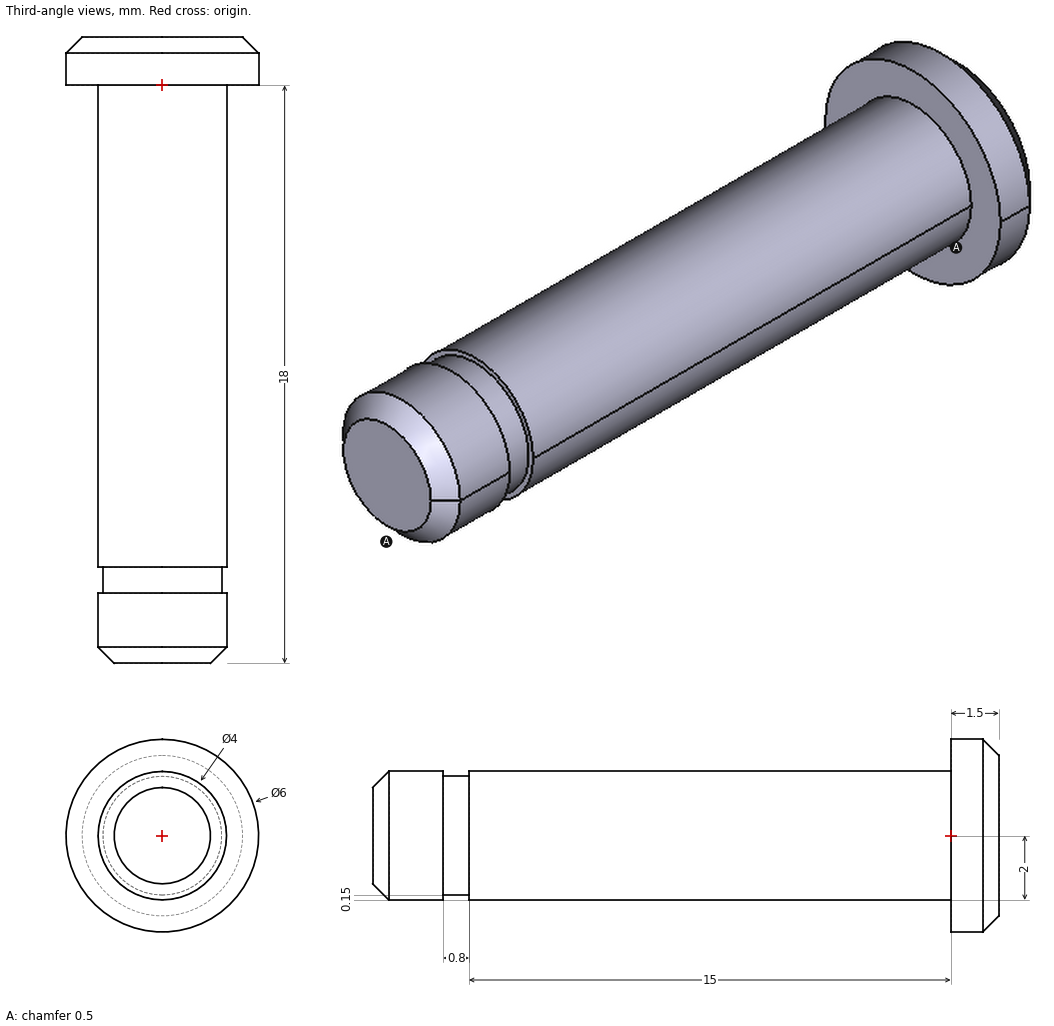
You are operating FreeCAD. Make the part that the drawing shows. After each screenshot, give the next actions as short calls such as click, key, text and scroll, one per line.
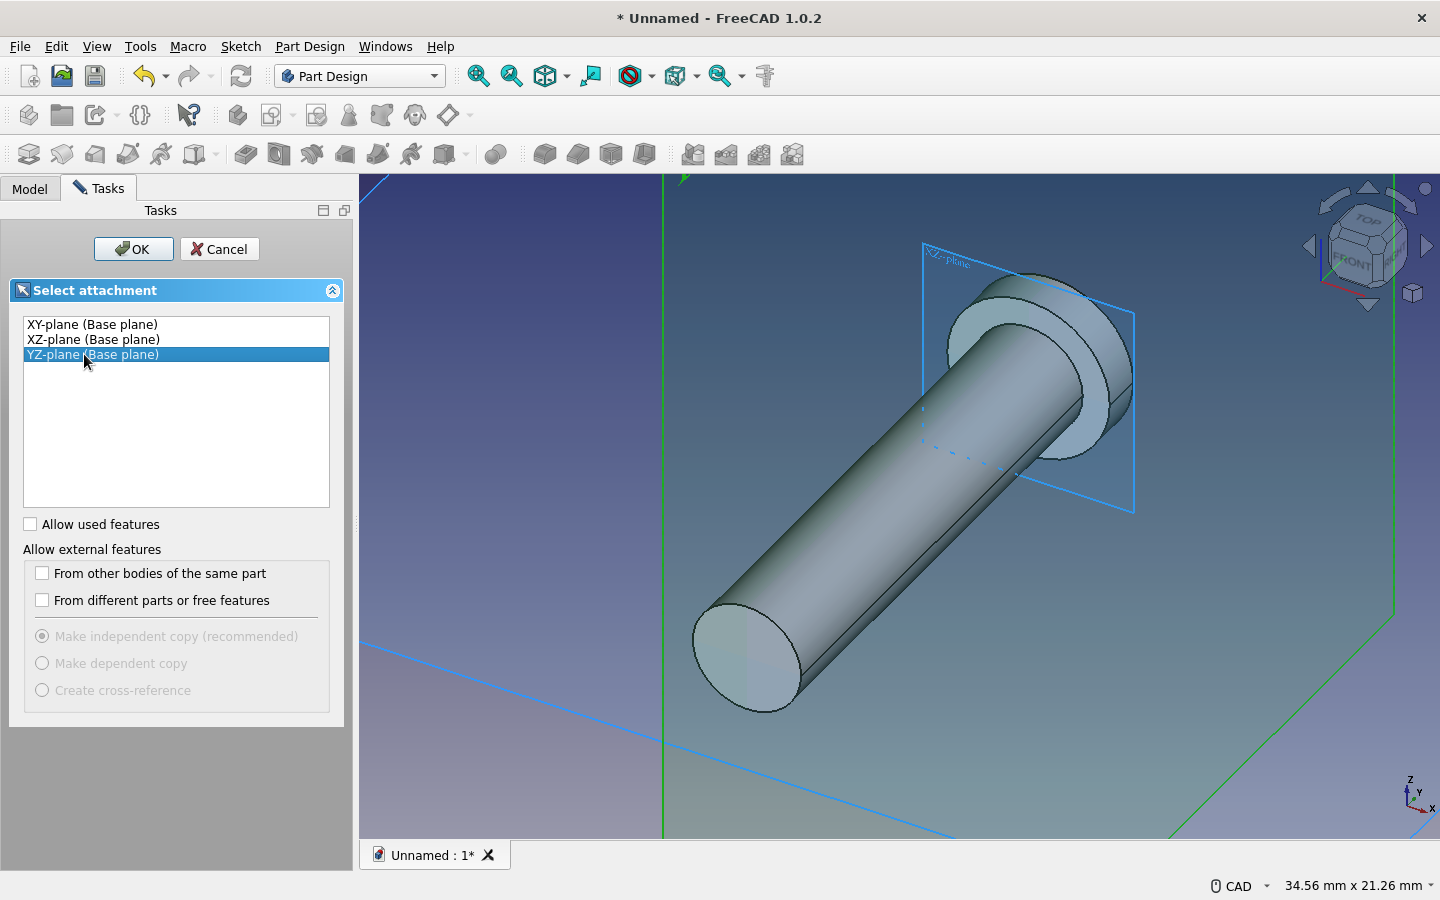
click(134, 249)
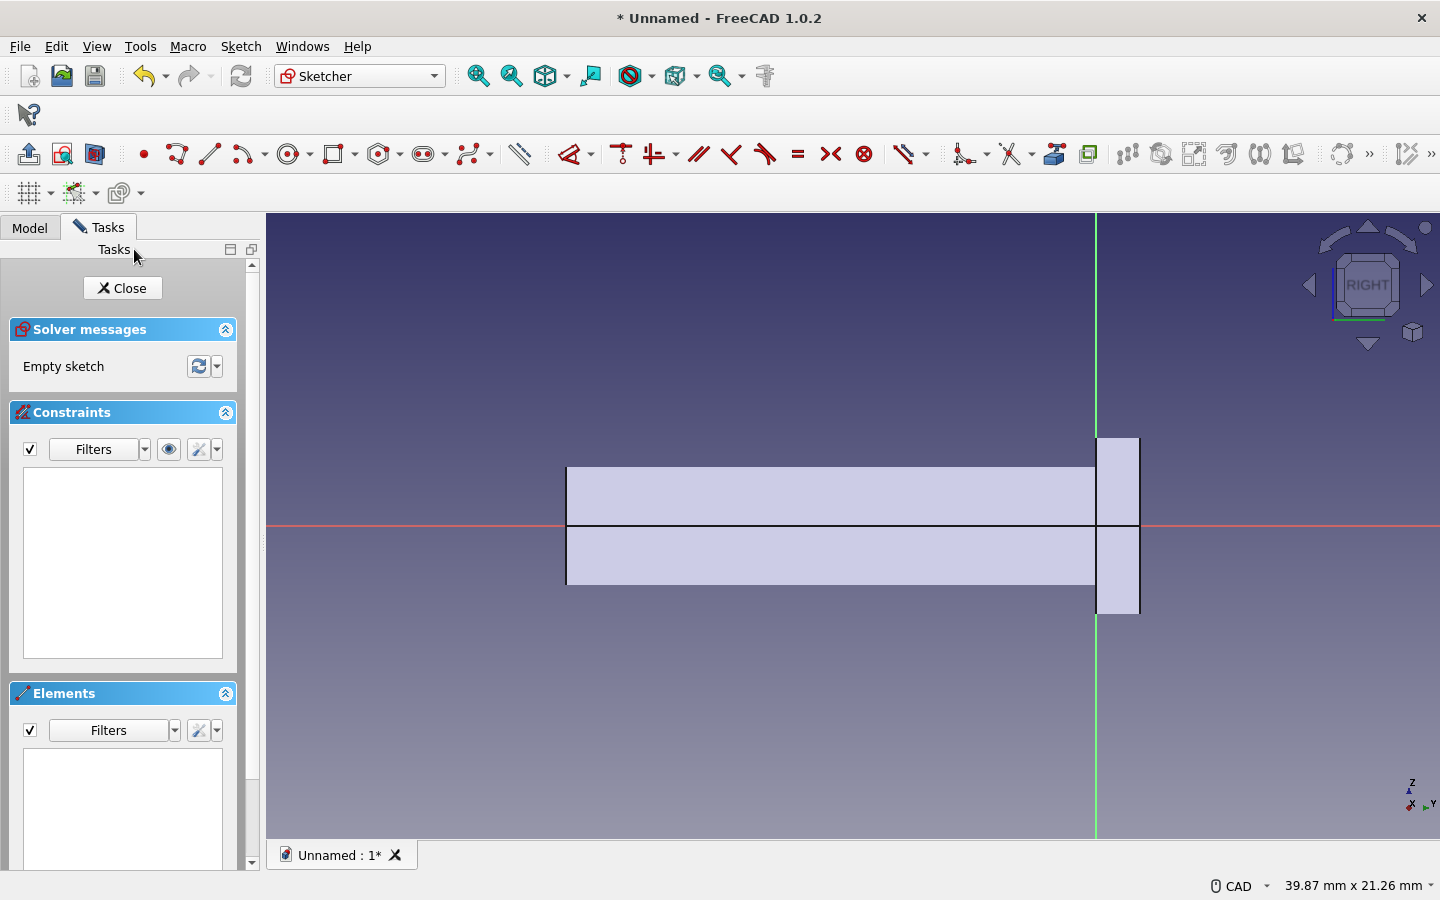
click(95, 154)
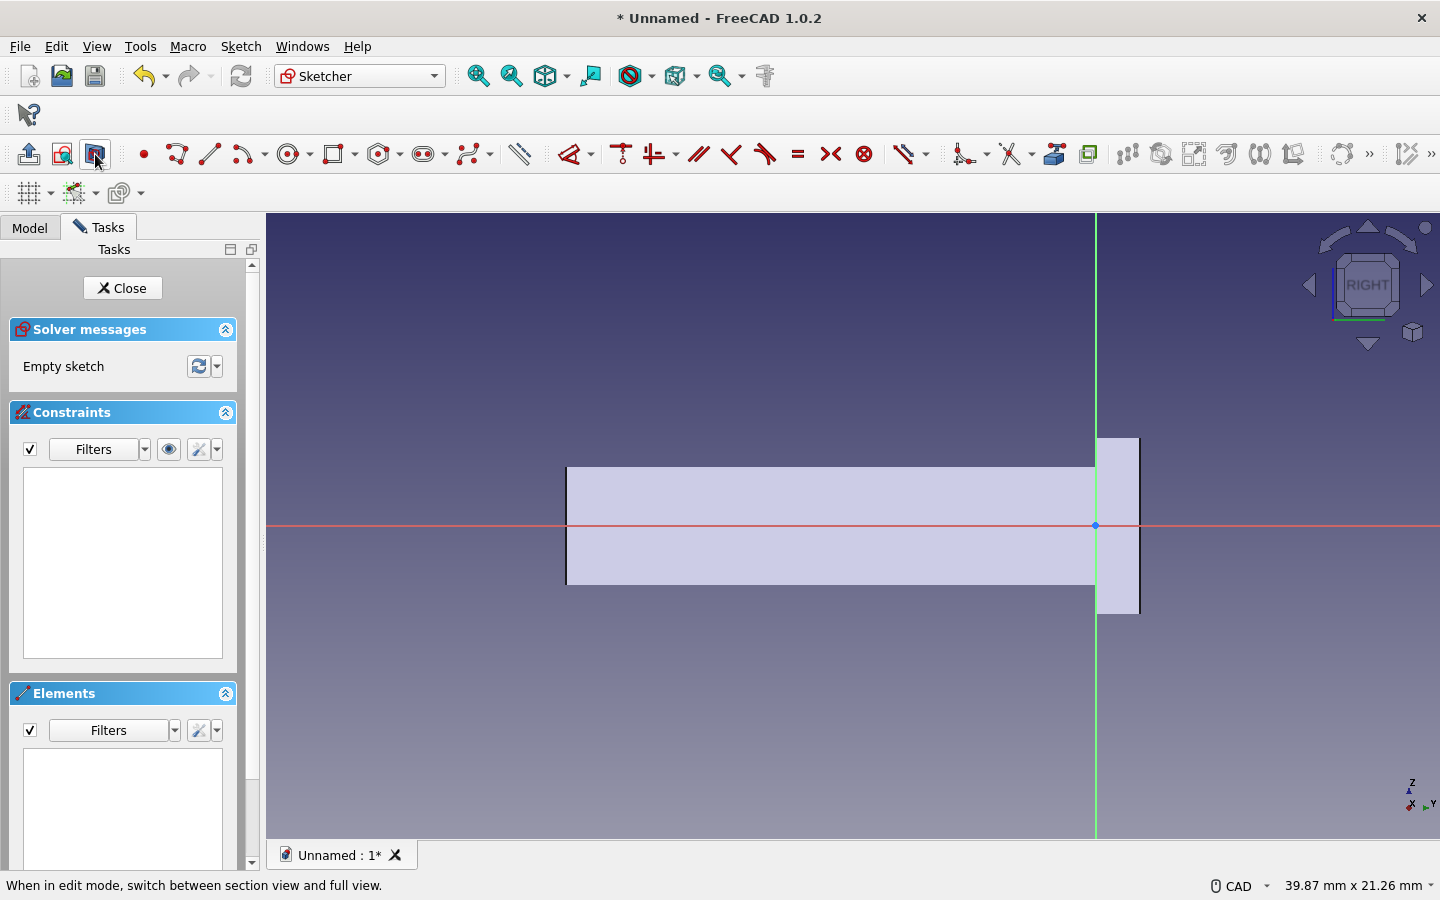
scroll(635, 586, up, 15)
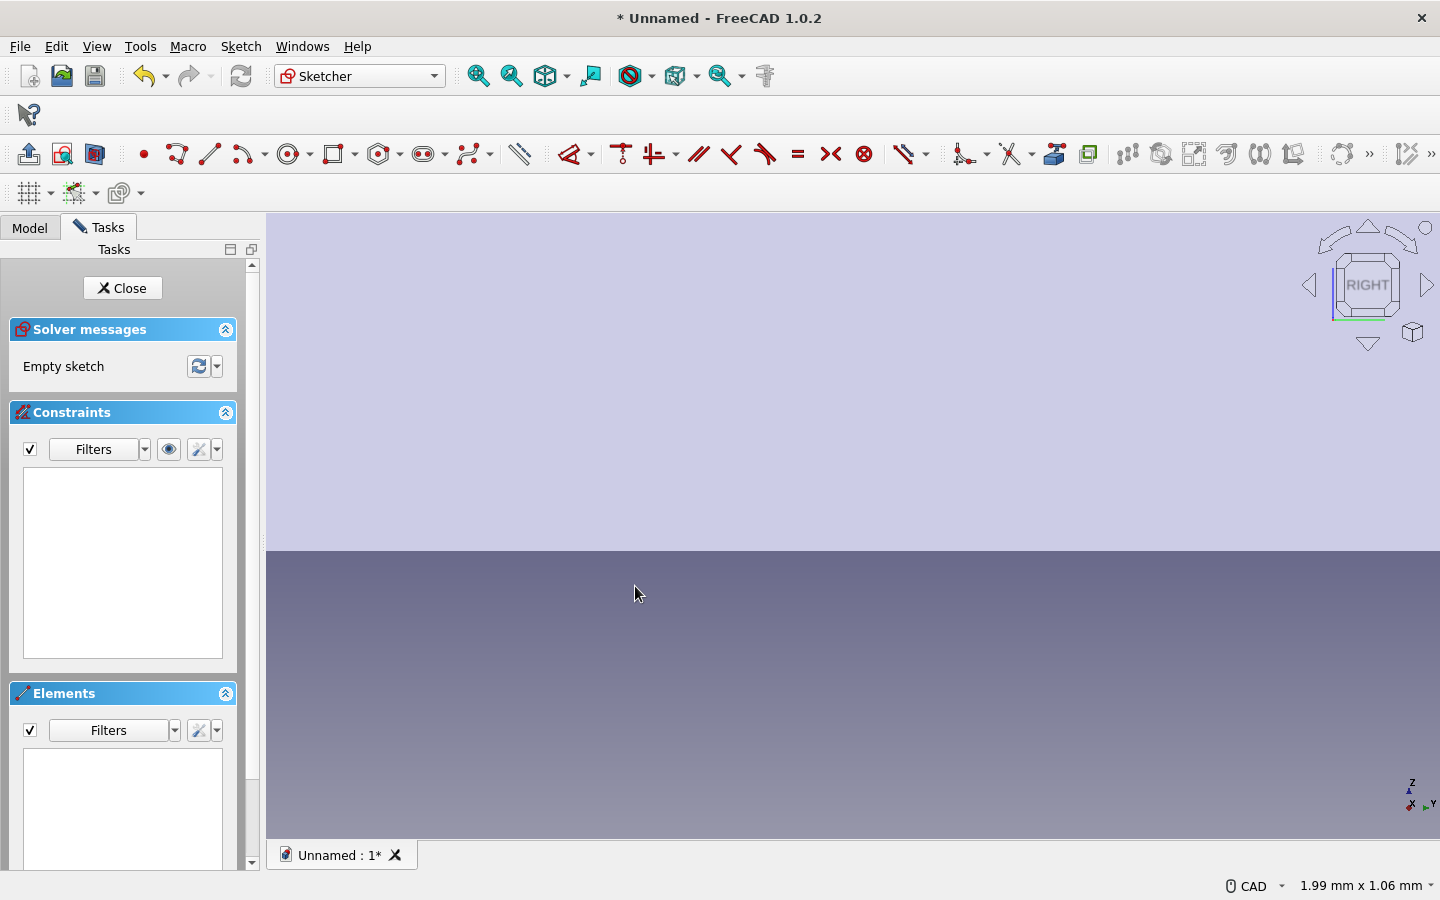
scroll(768, 471, up, 2)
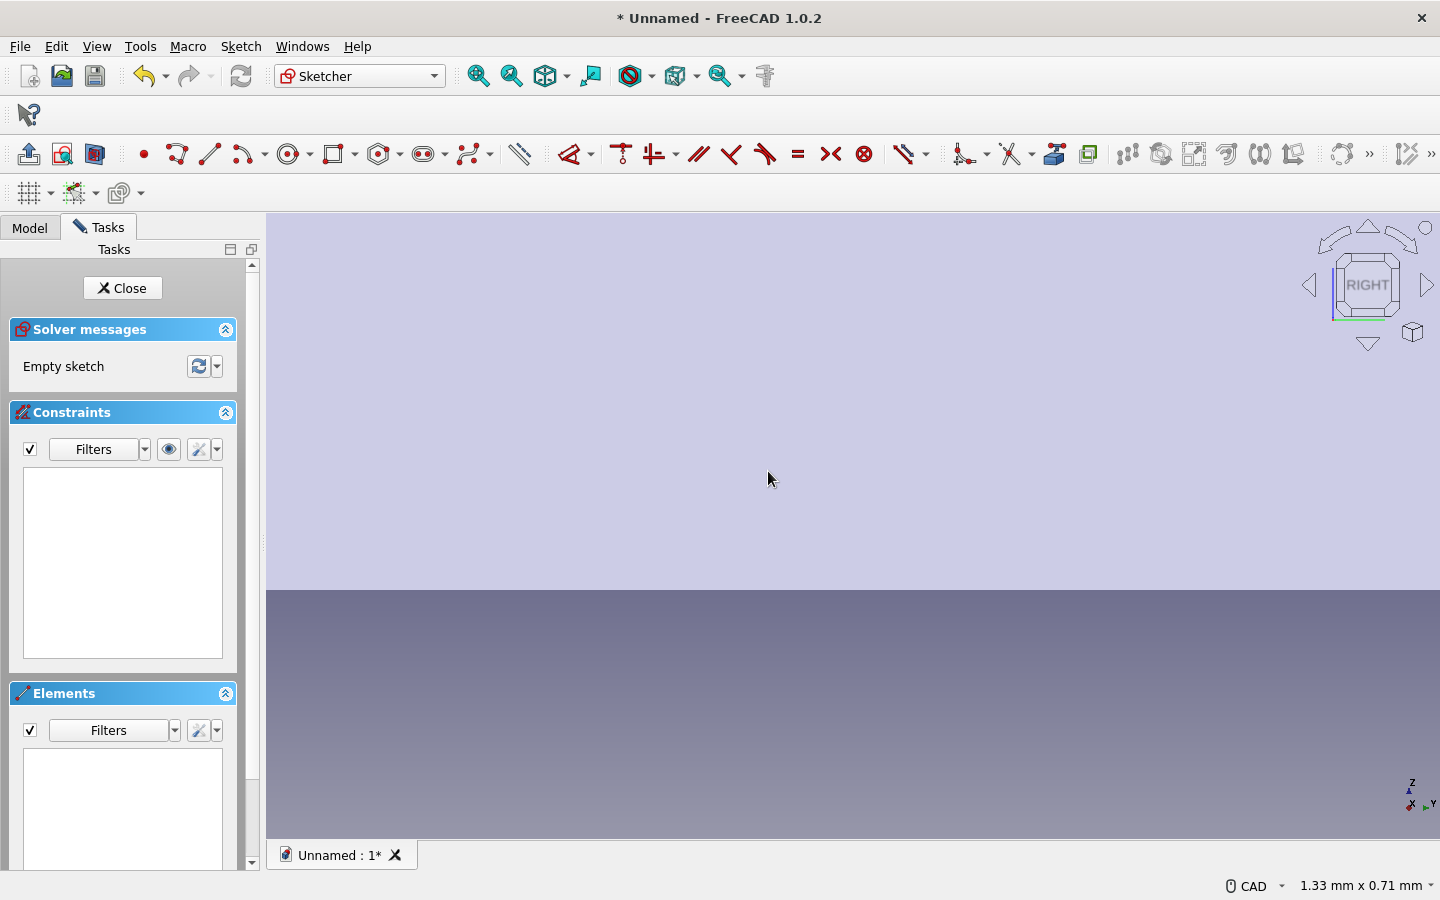
click(332, 154)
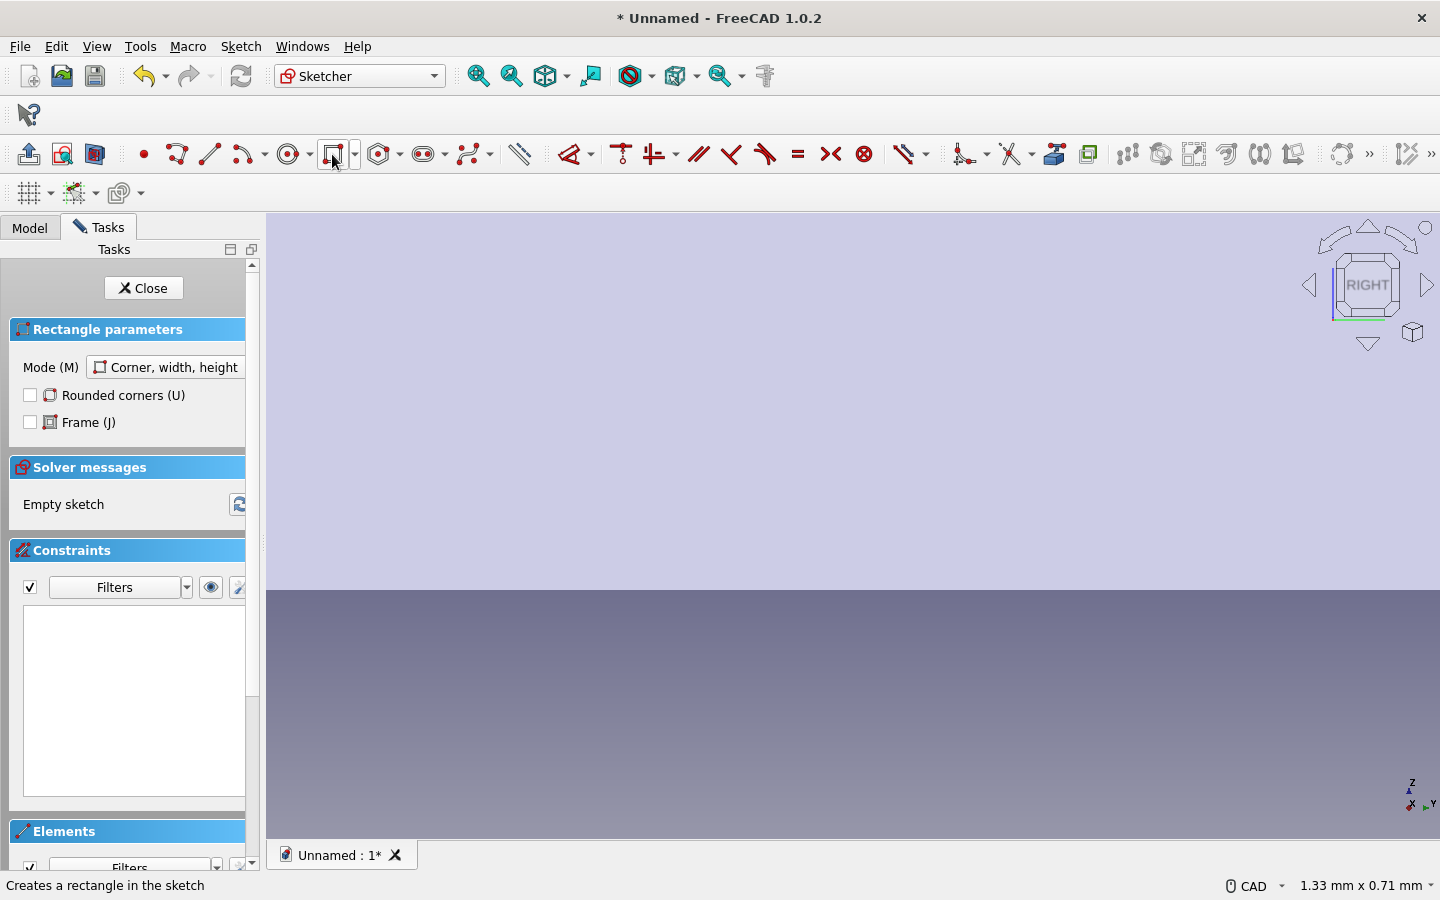
click(431, 460)
click(1137, 592)
key(Escape)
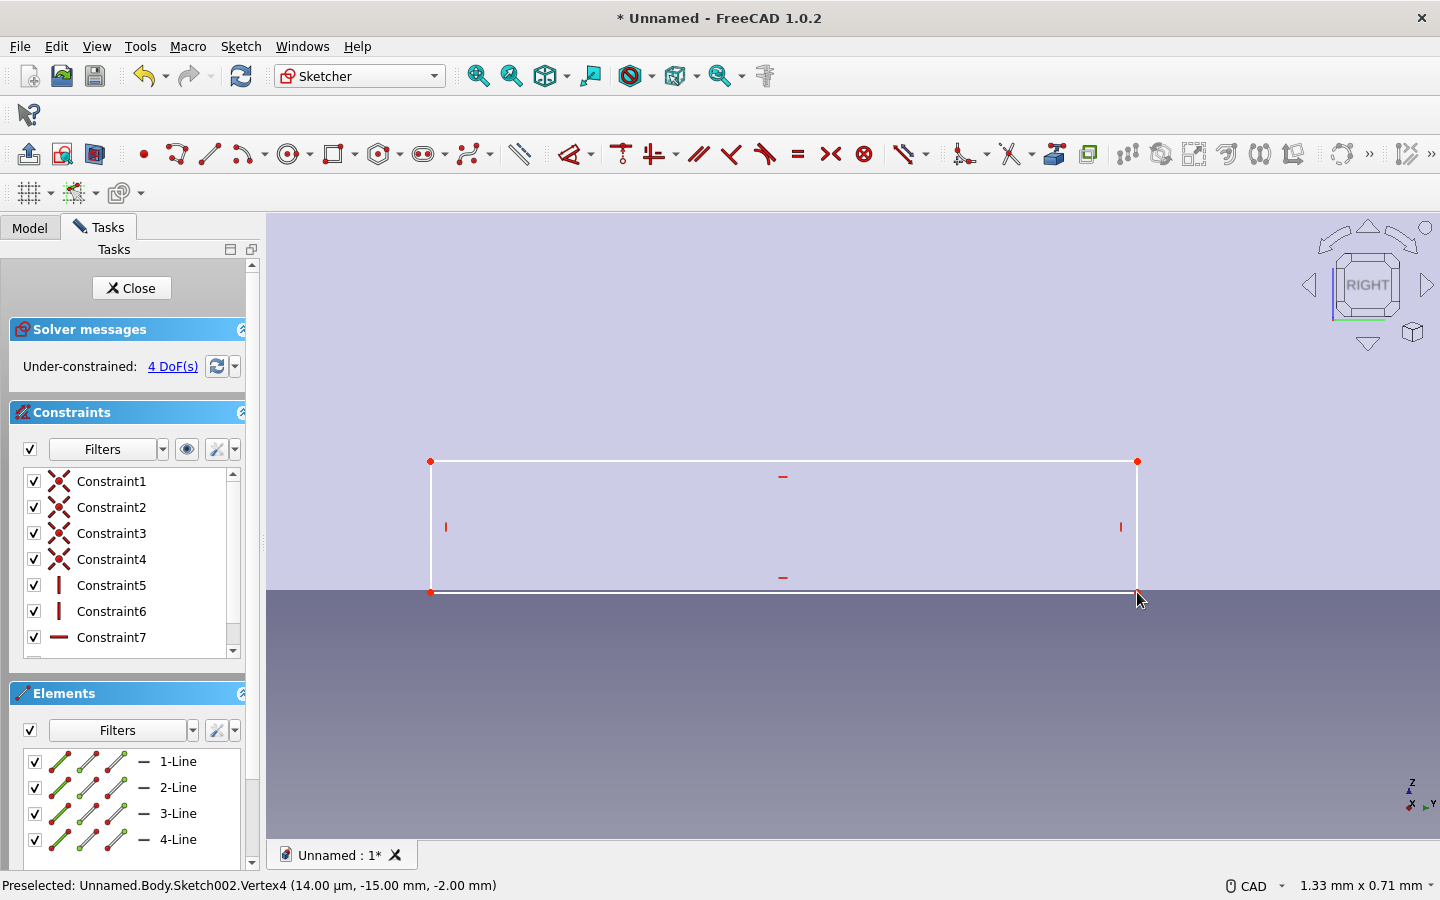
click(568, 154)